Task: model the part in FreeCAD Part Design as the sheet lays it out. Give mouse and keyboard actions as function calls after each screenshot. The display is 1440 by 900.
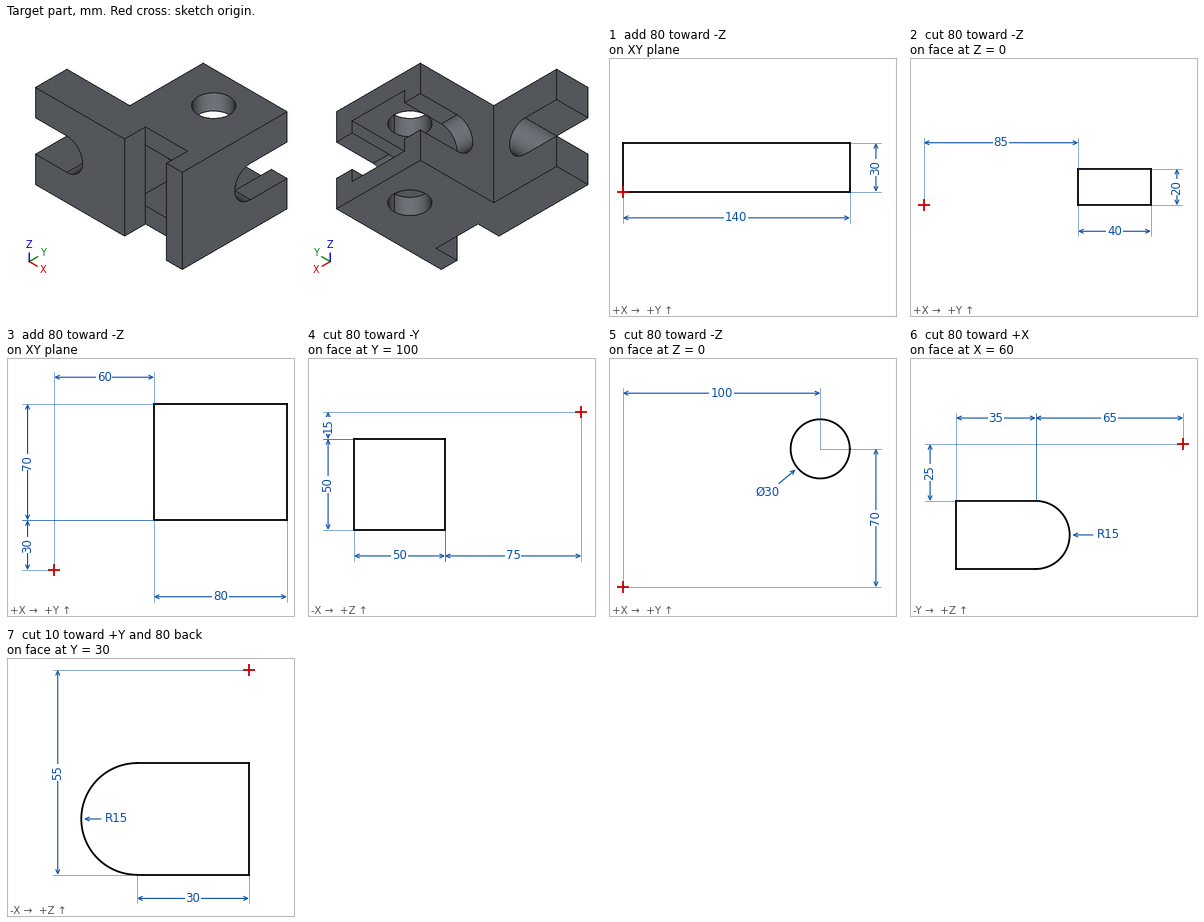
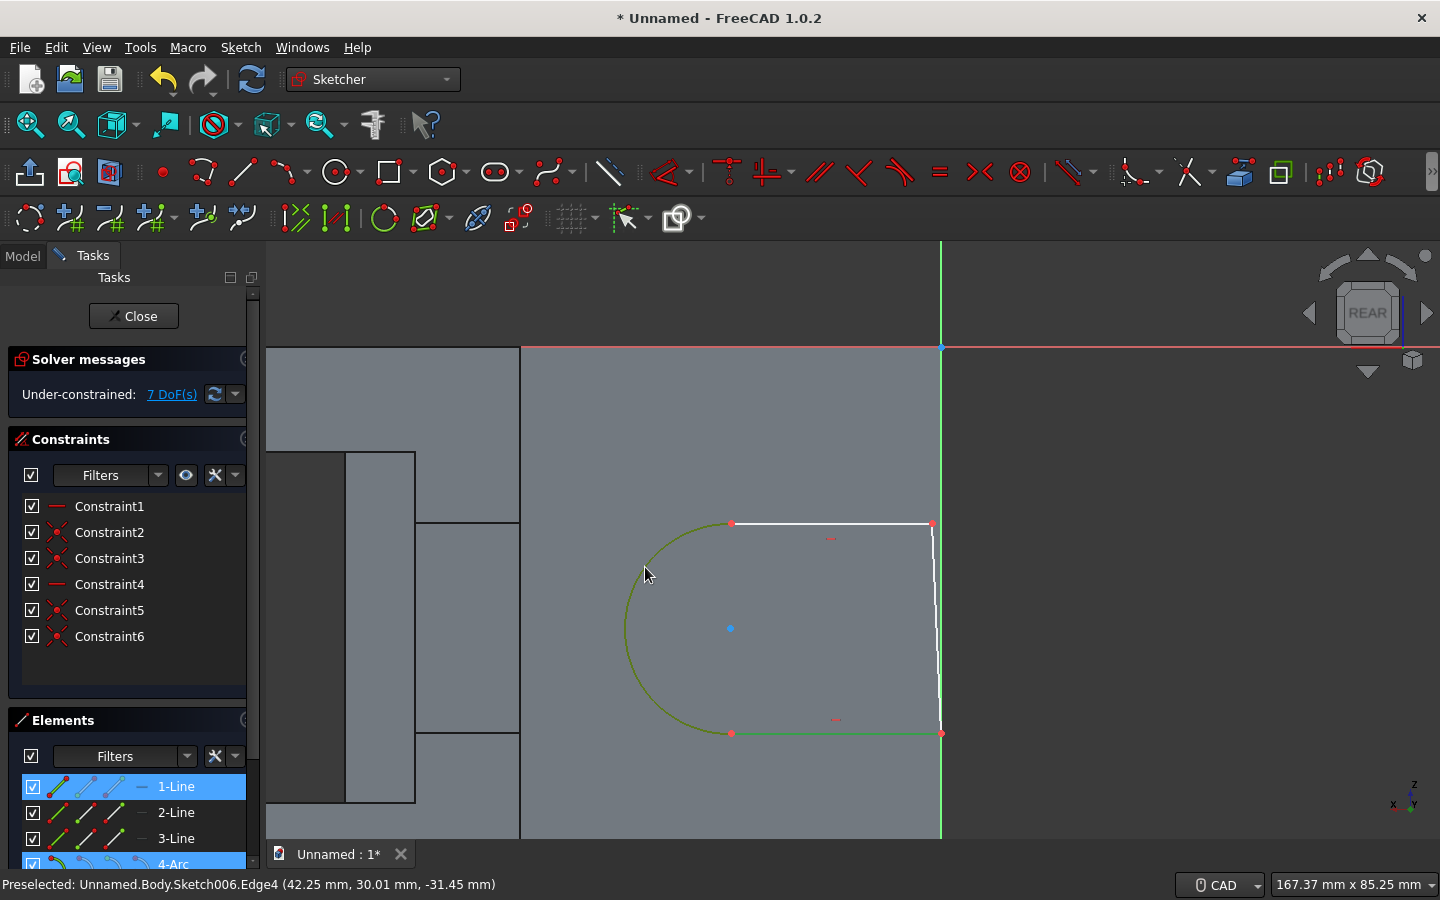
key(t)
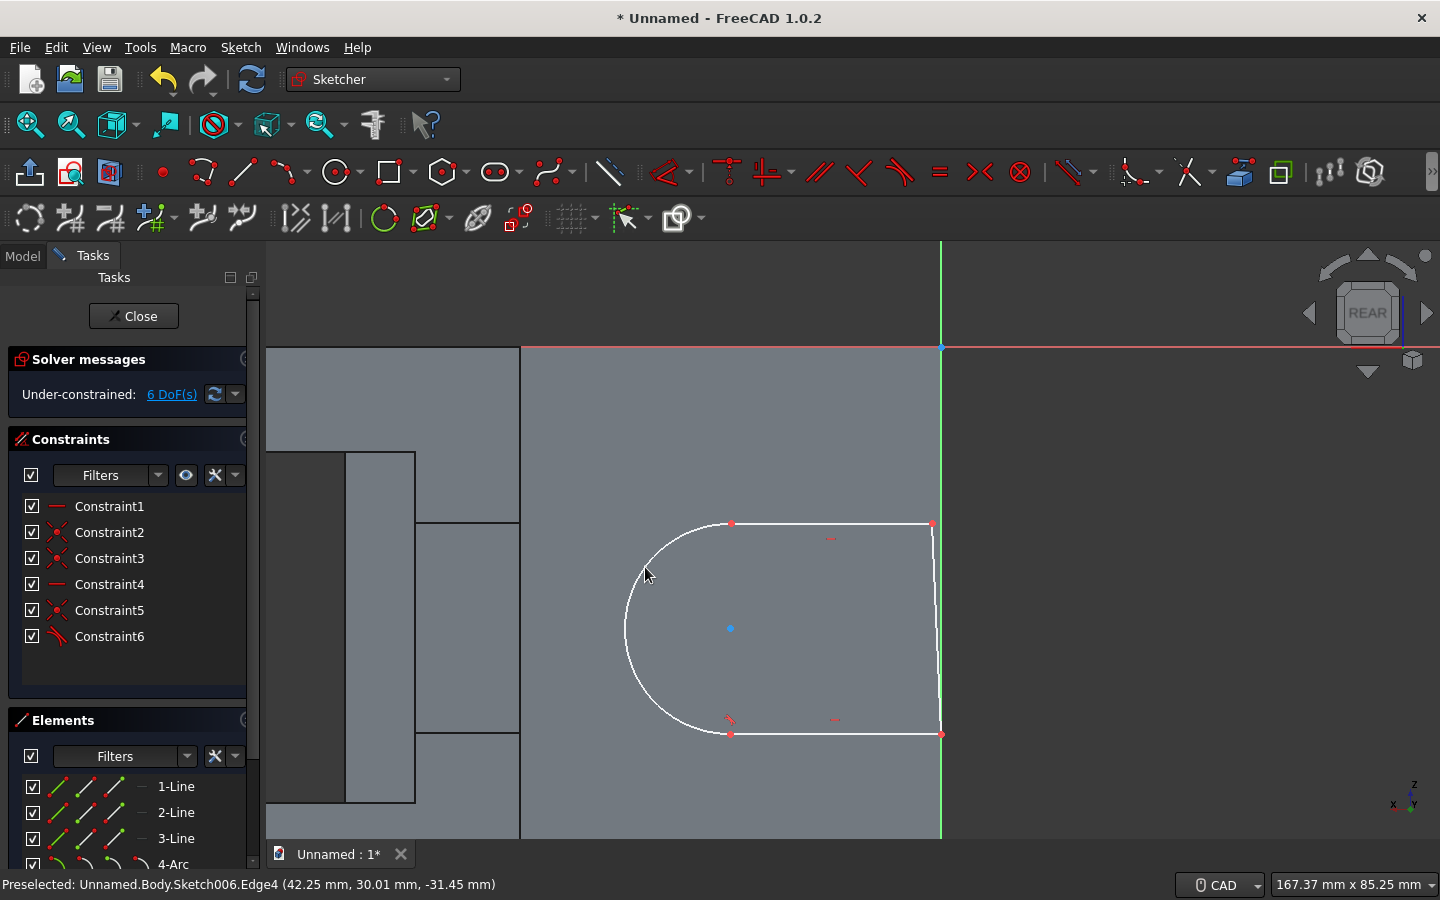
click(872, 524)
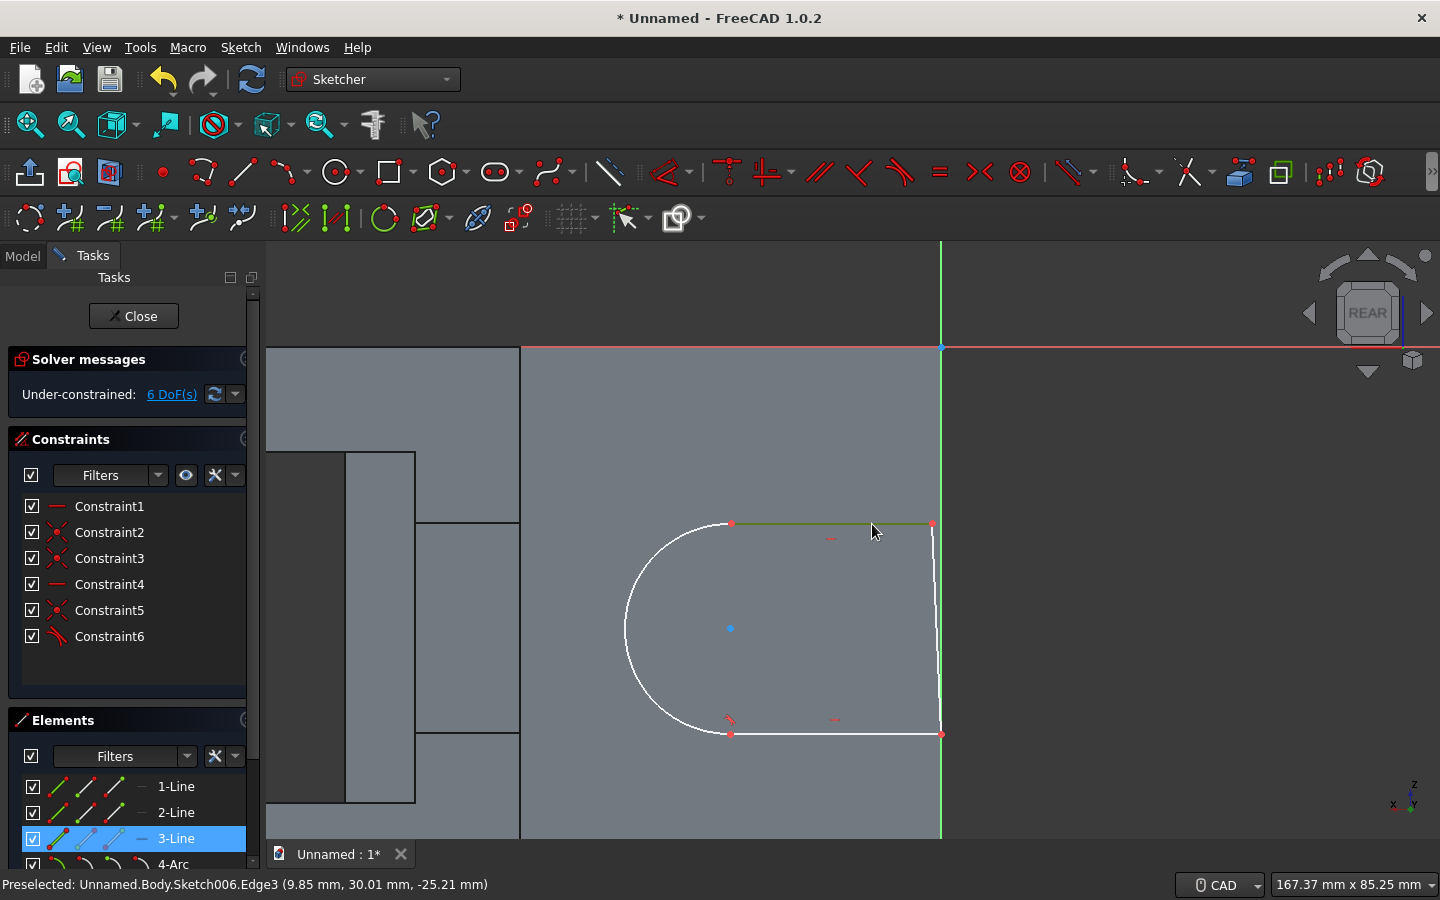
click(645, 567)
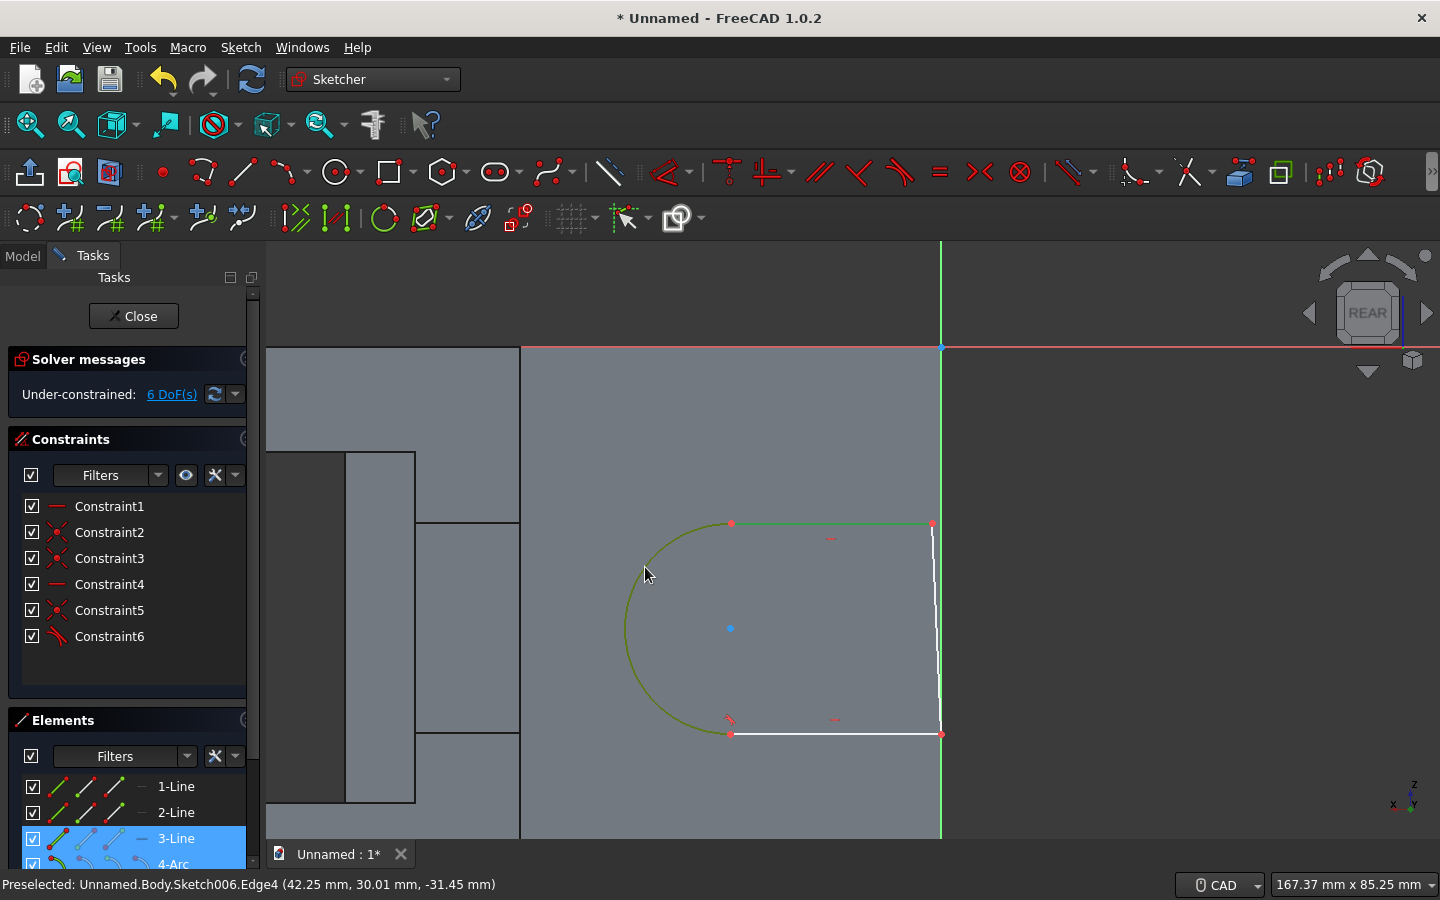
click(900, 172)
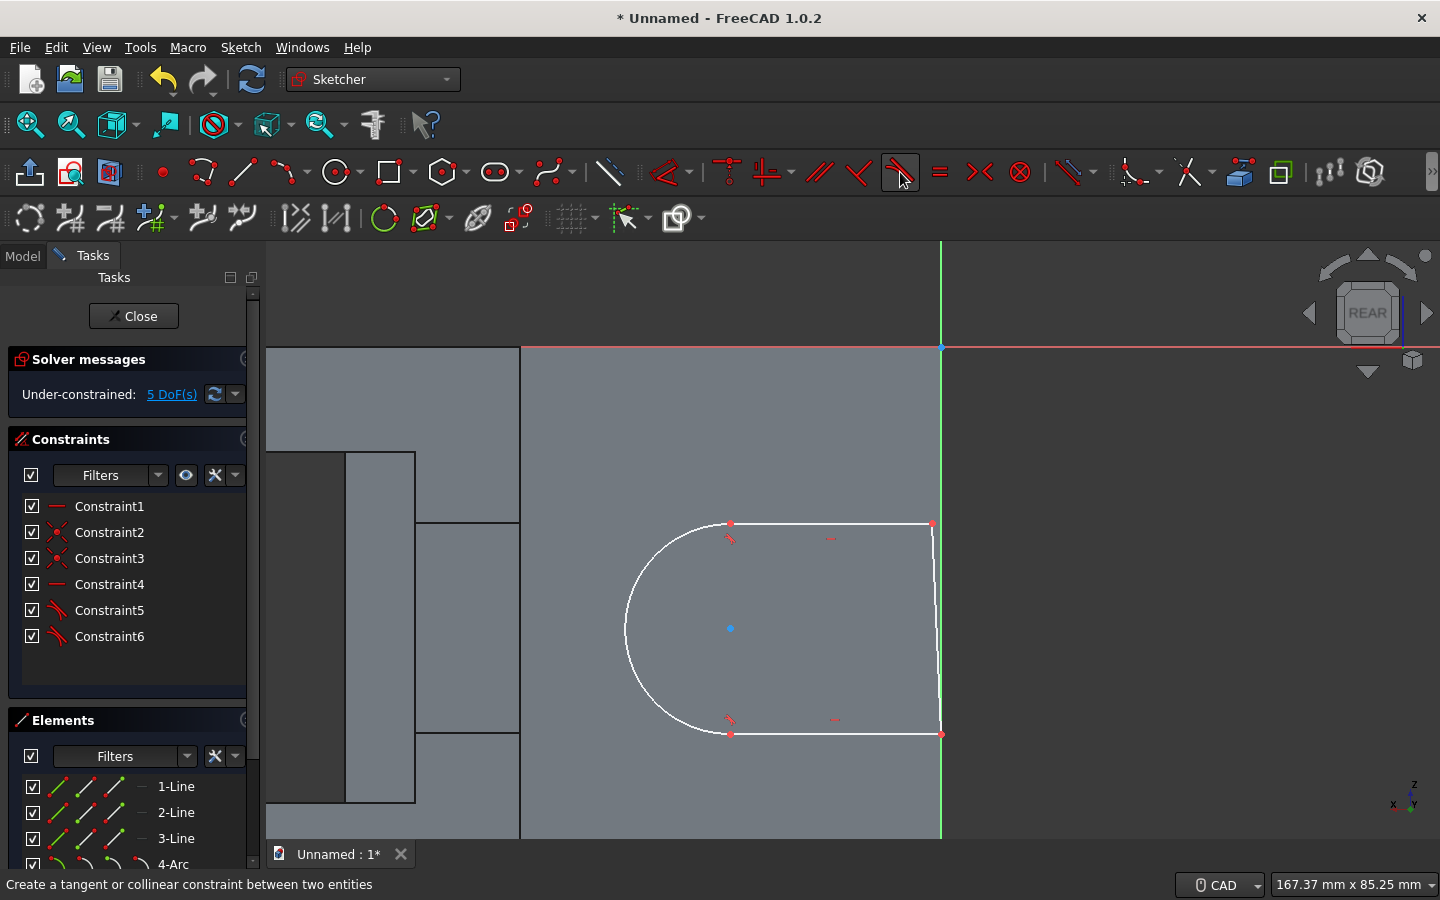
click(938, 671)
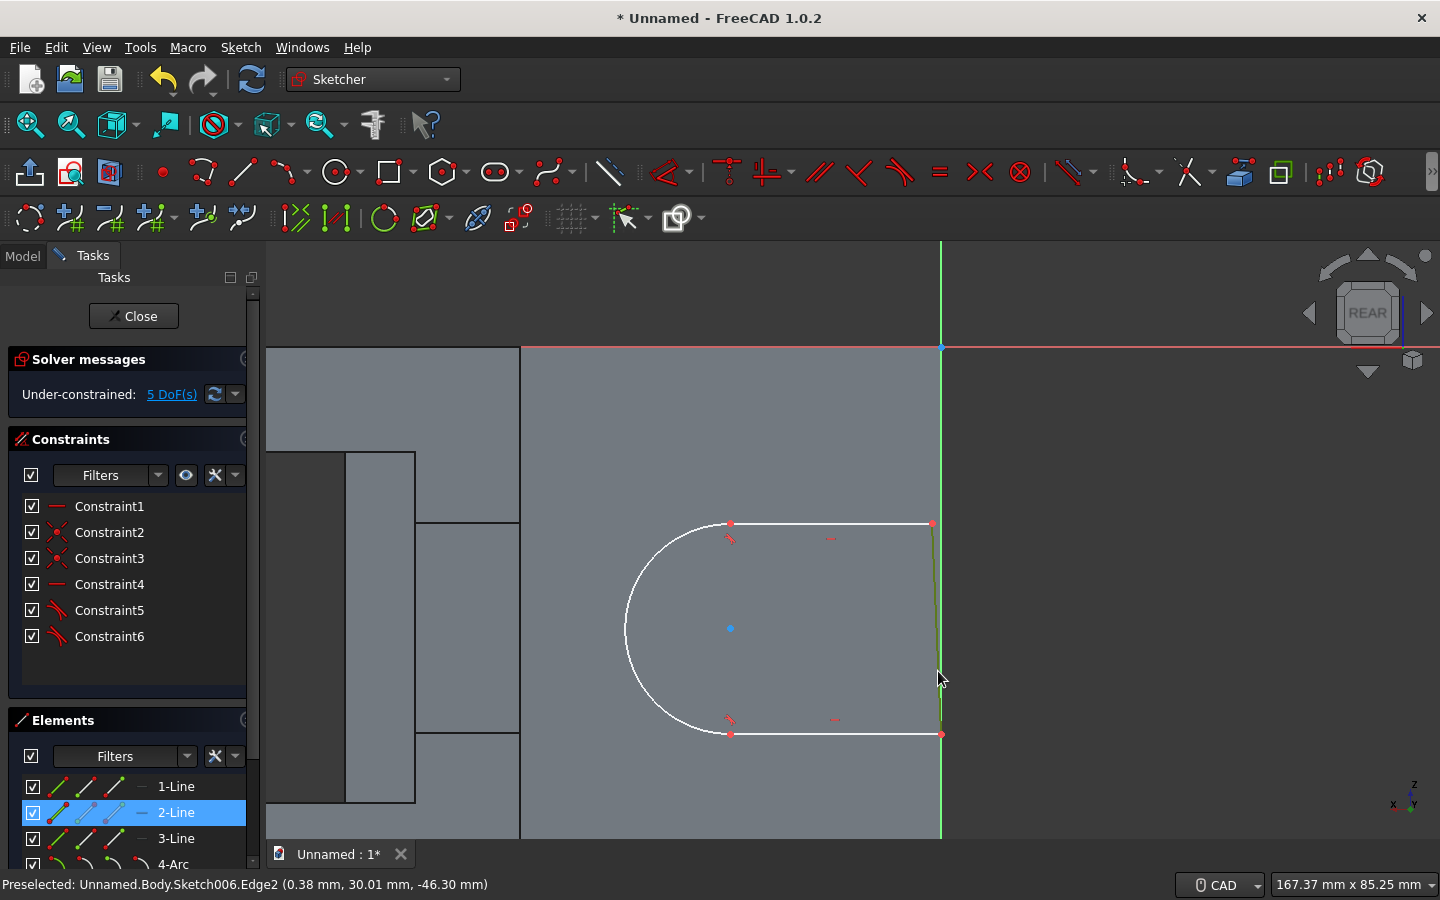
key(v)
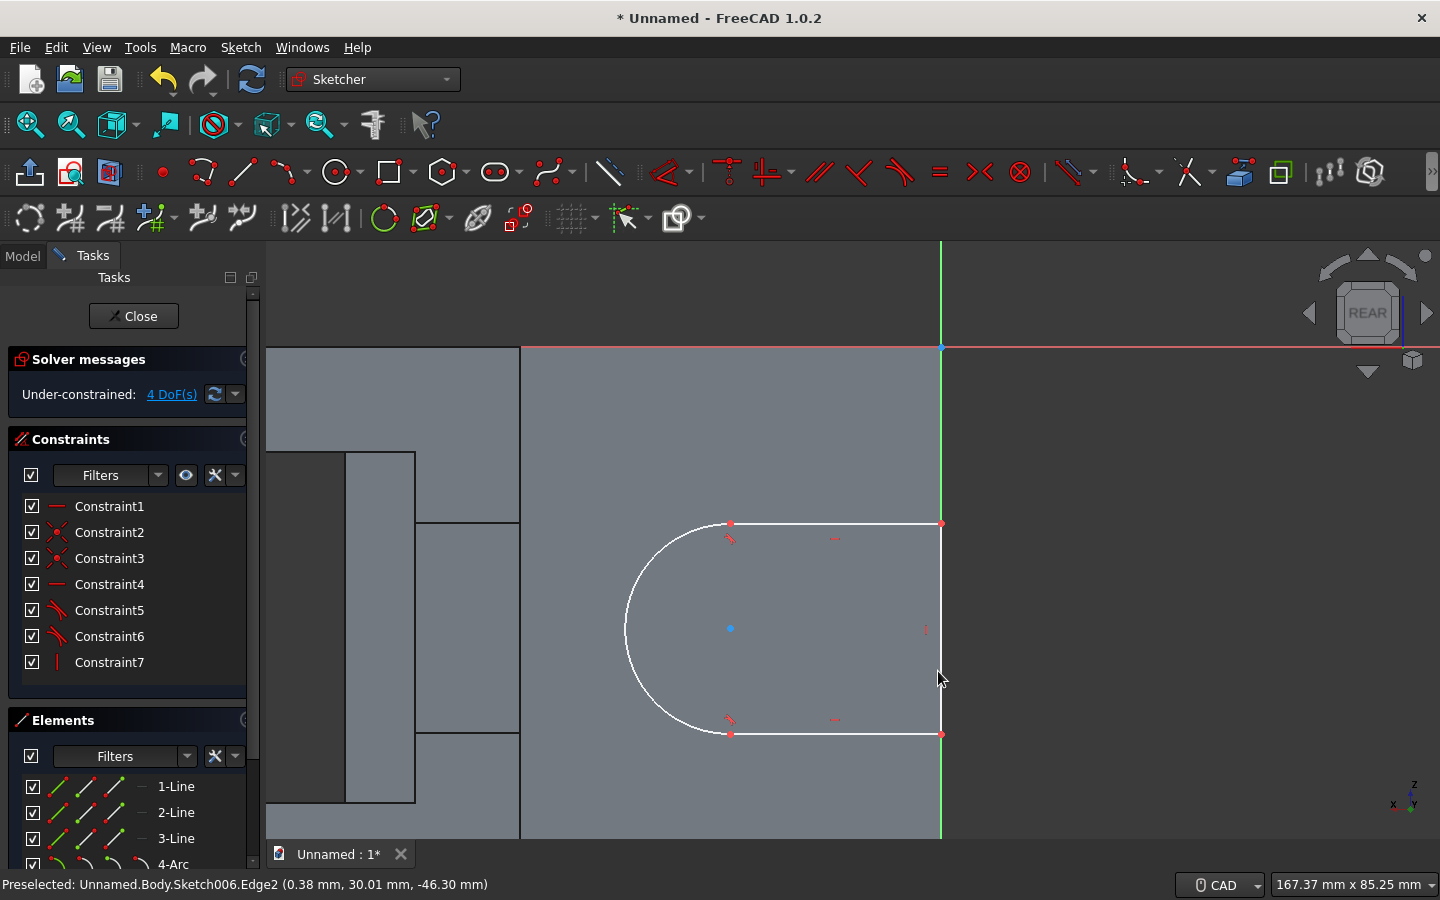
key(d)